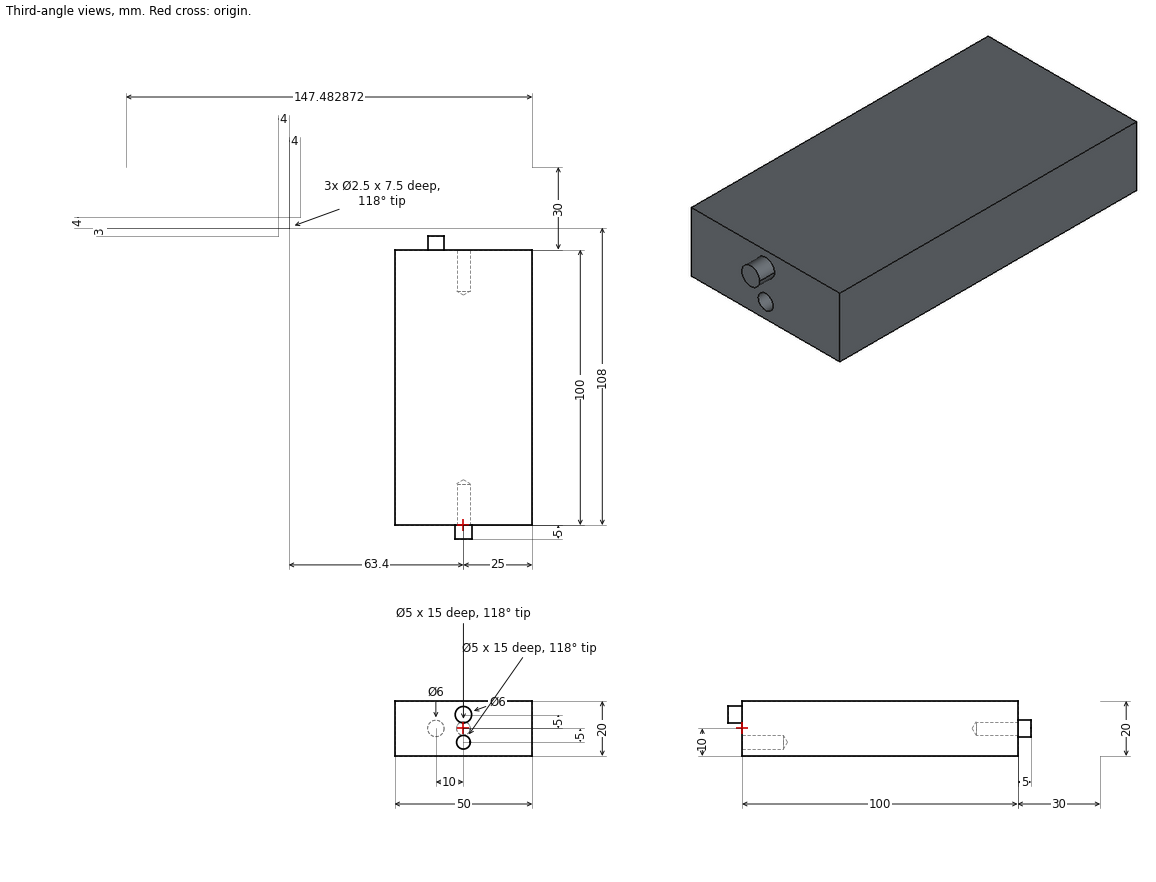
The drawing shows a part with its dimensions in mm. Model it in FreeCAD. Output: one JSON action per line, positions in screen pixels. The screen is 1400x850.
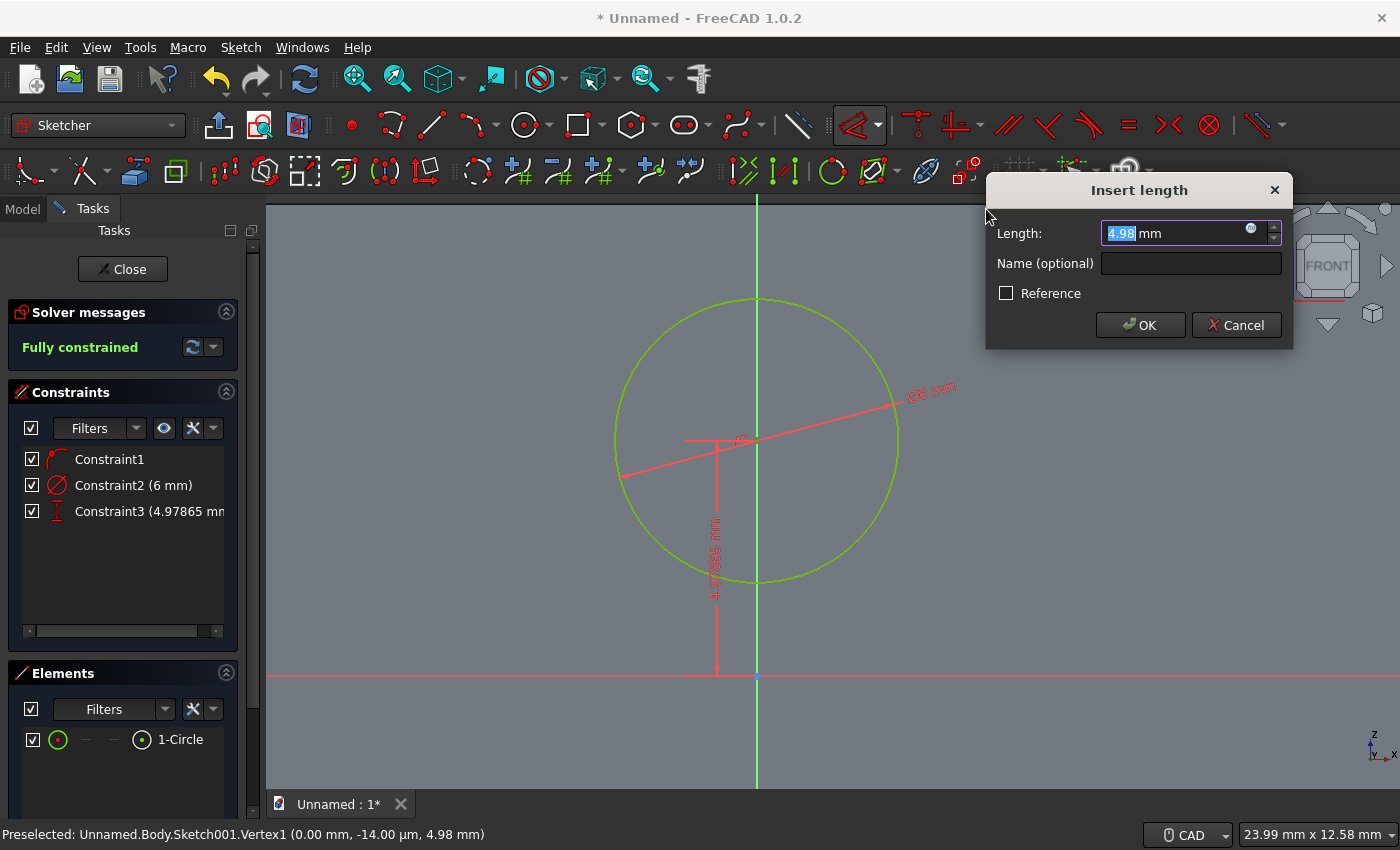
{"action": "type", "text": "5"}
{"action": "key", "text": "Return"}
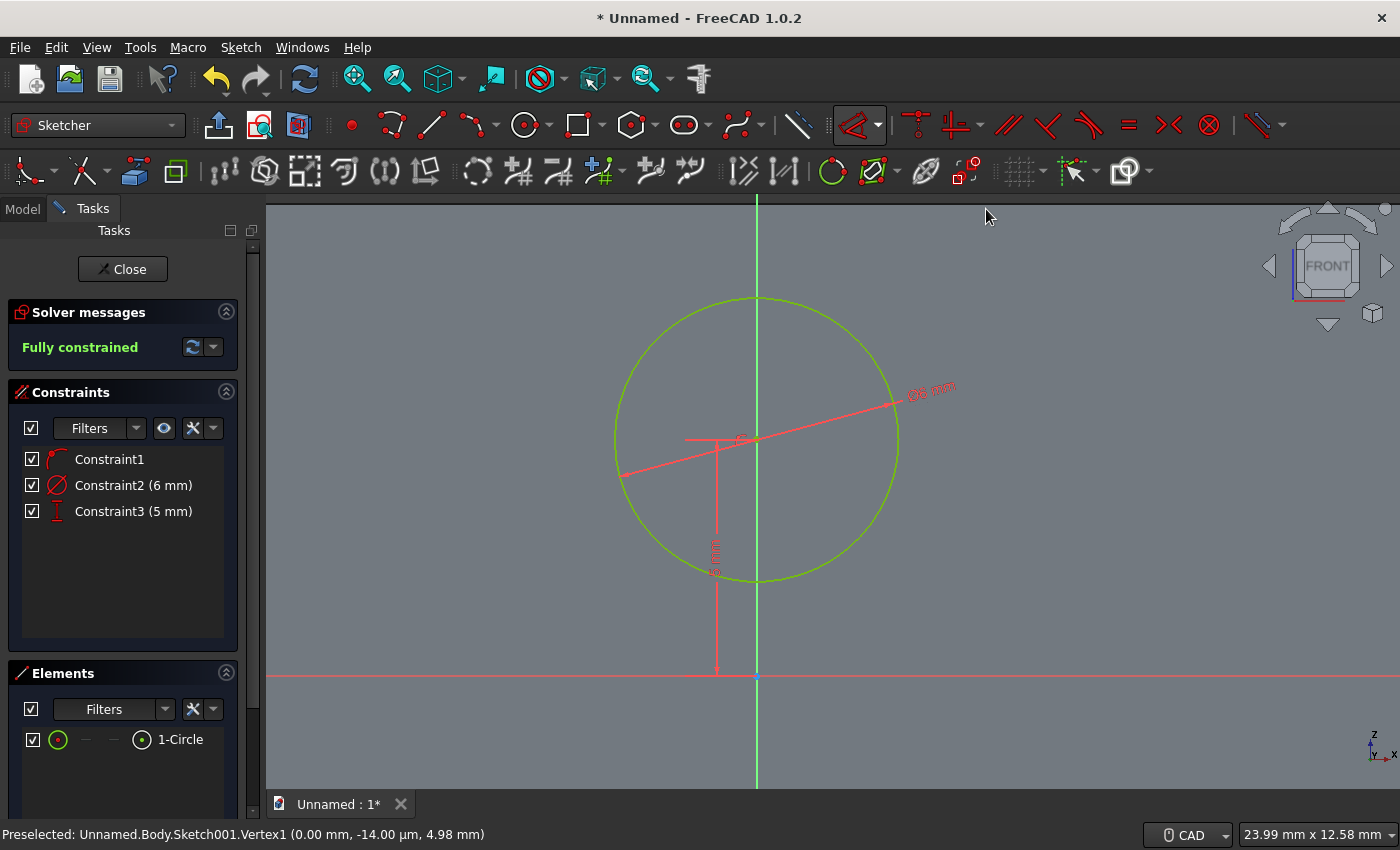
{"action": "left_click", "coordinate": [123, 269]}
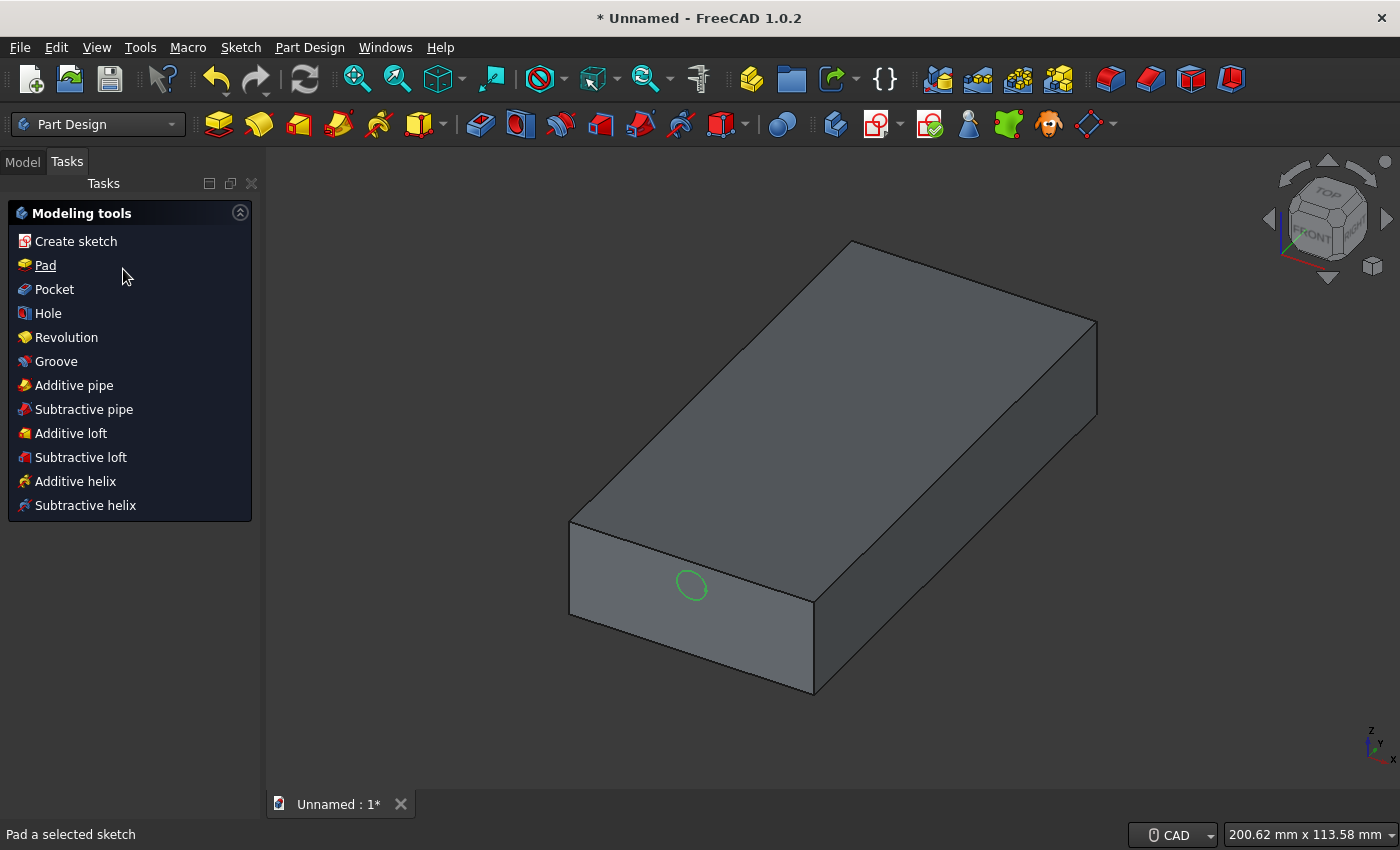
{"action": "left_click", "coordinate": [220, 124]}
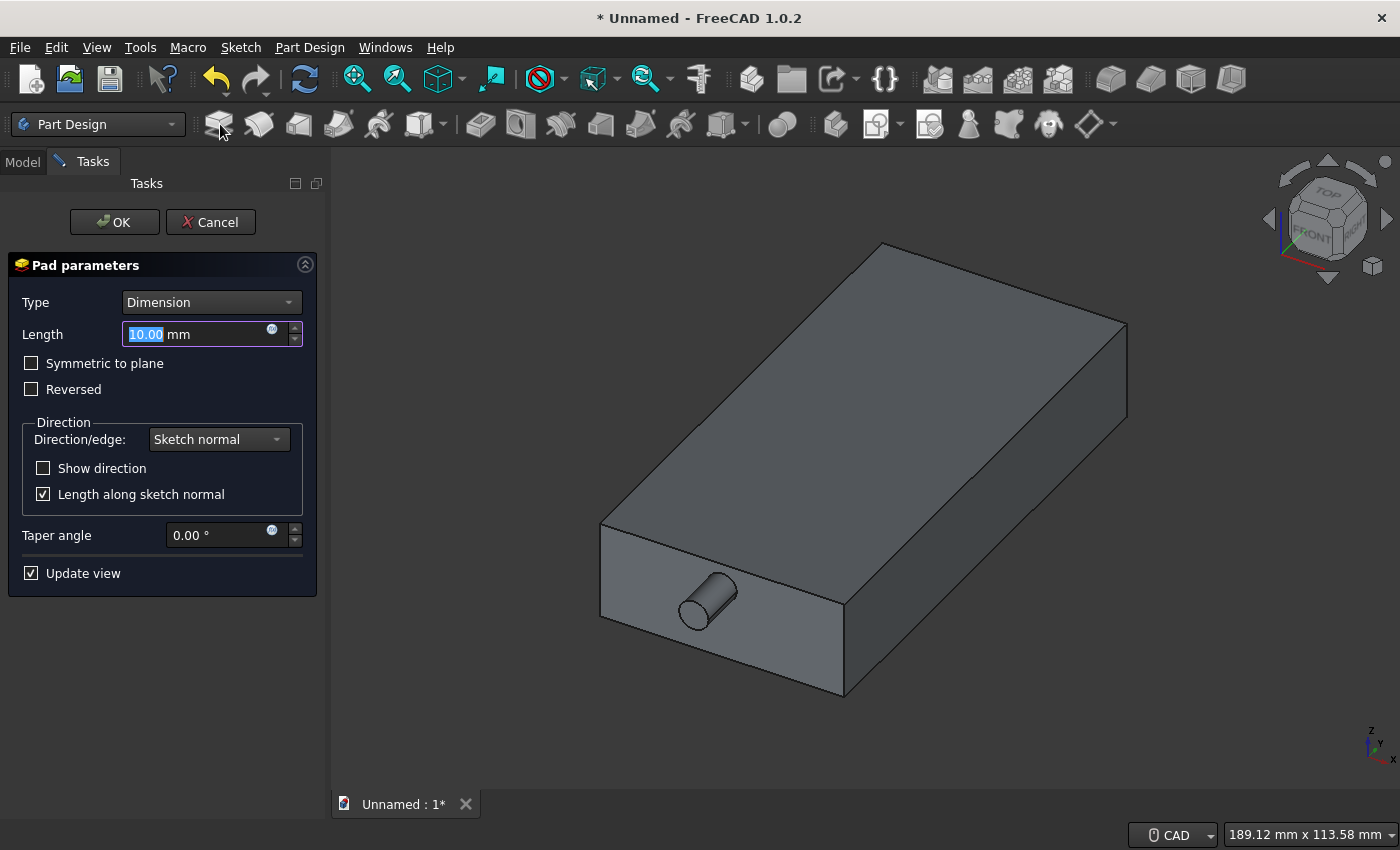
{"action": "type", "text": "5"}
{"action": "key", "text": "Tab"}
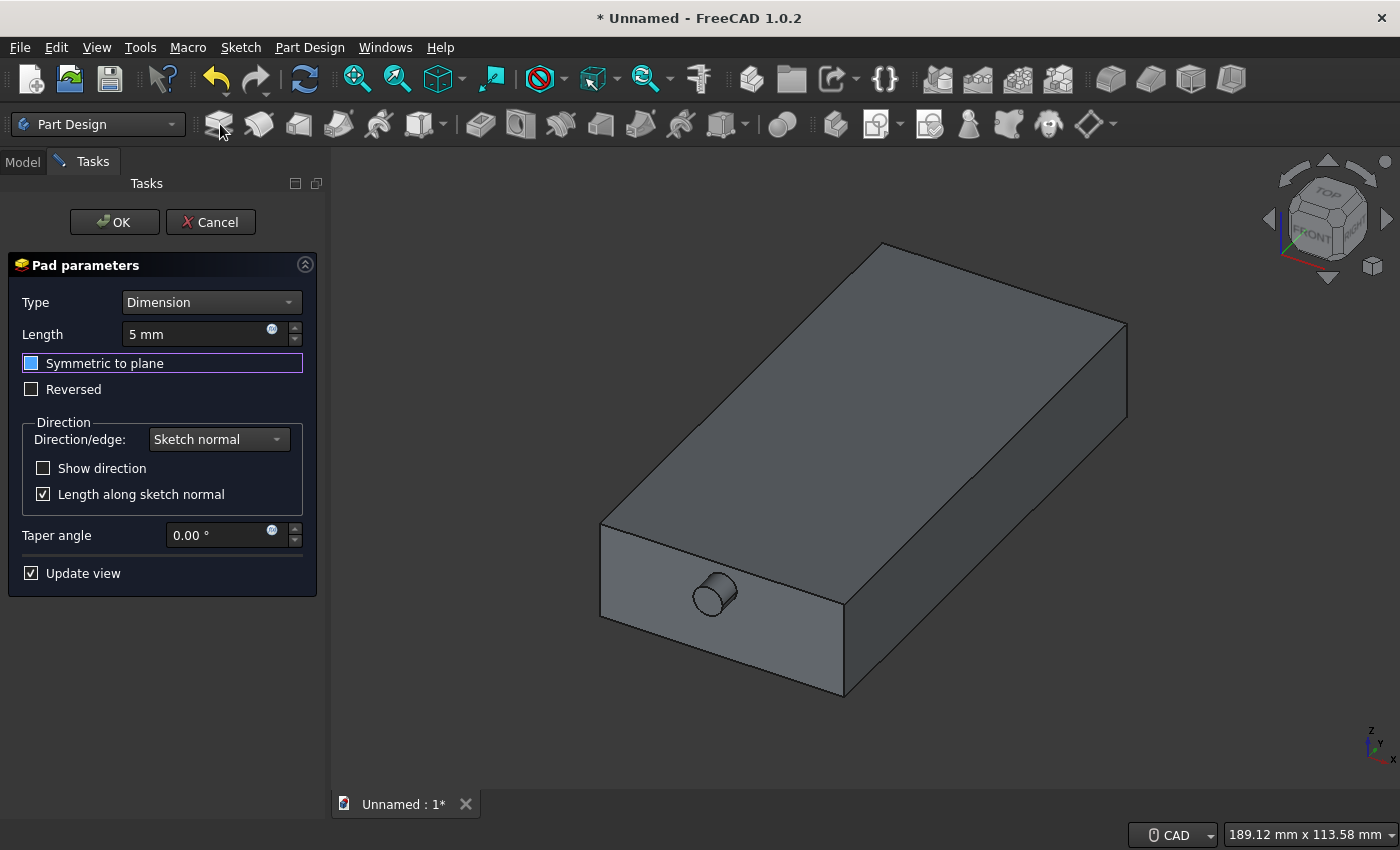
{"action": "left_click", "coordinate": [115, 222]}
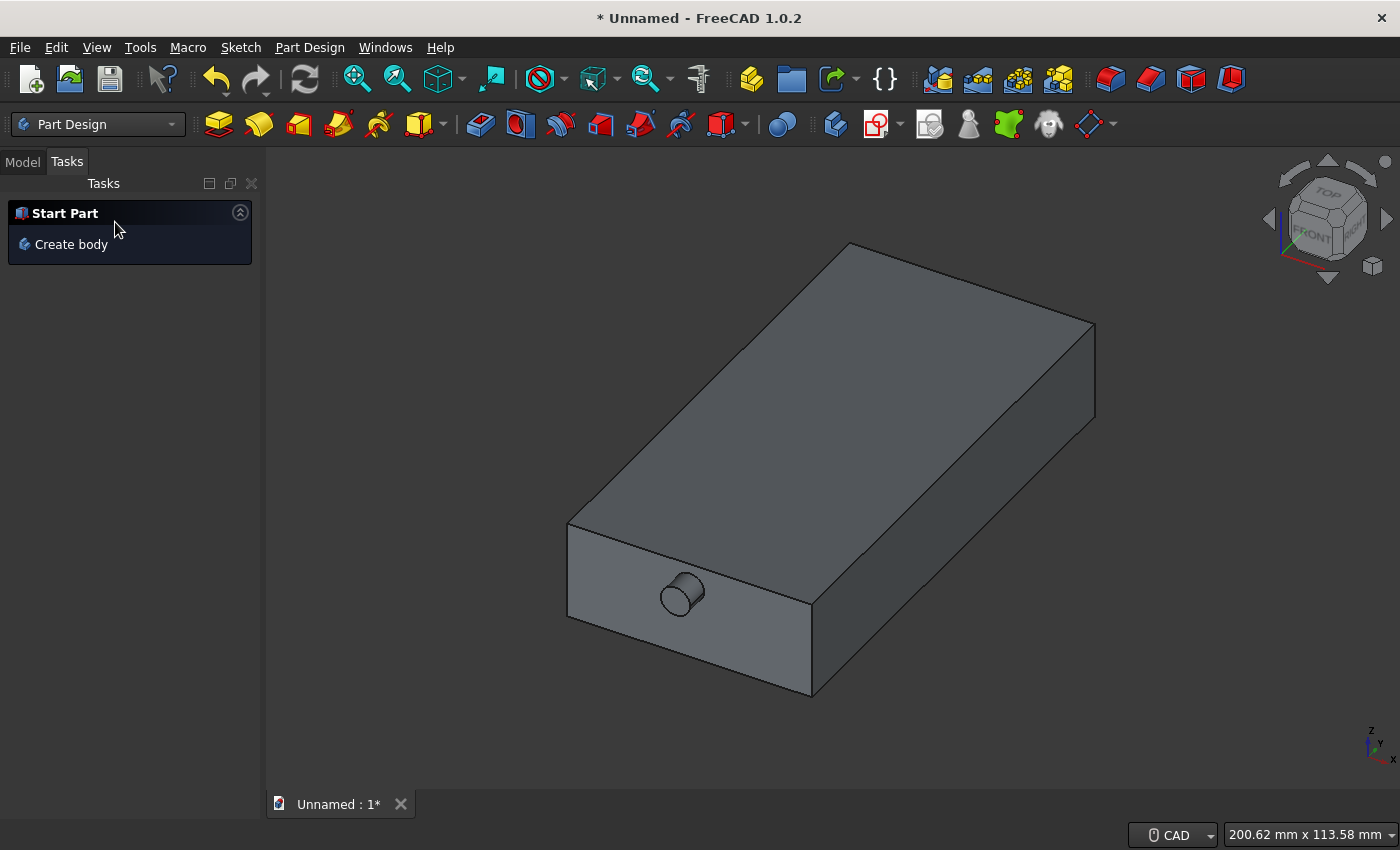
{"action": "left_click", "coordinate": [876, 124]}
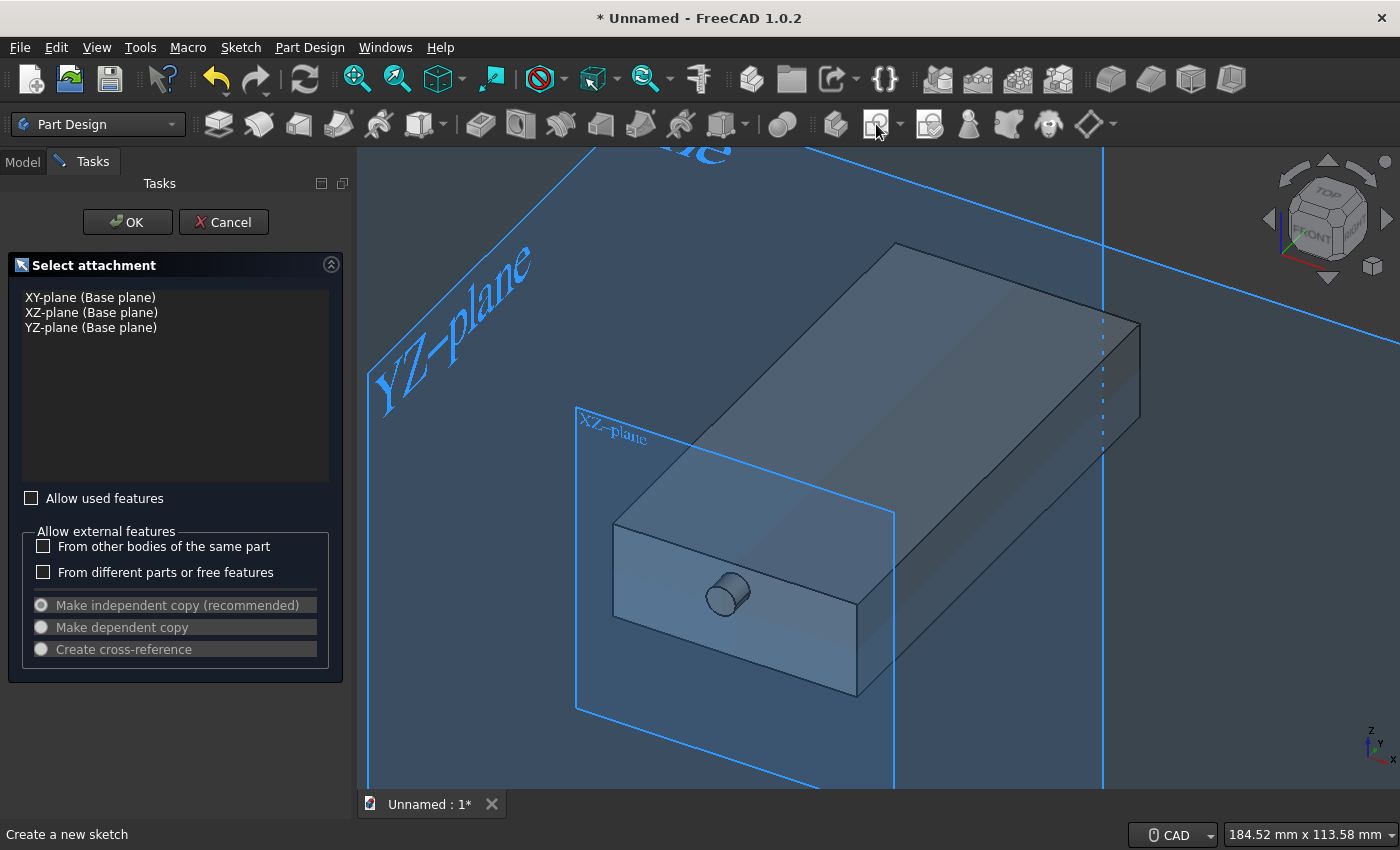
{"action": "left_click", "coordinate": [82, 312]}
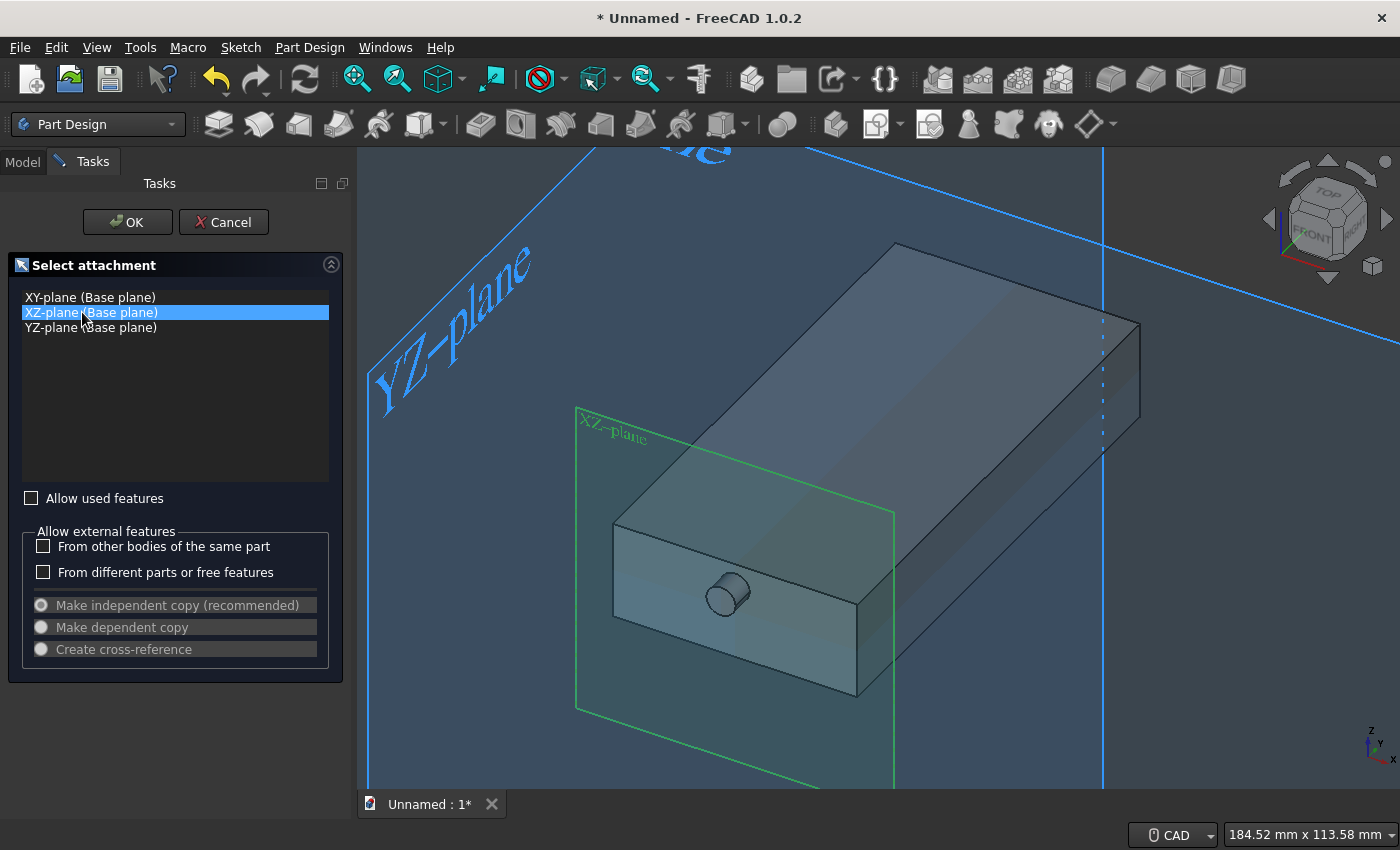
{"action": "left_click", "coordinate": [128, 222]}